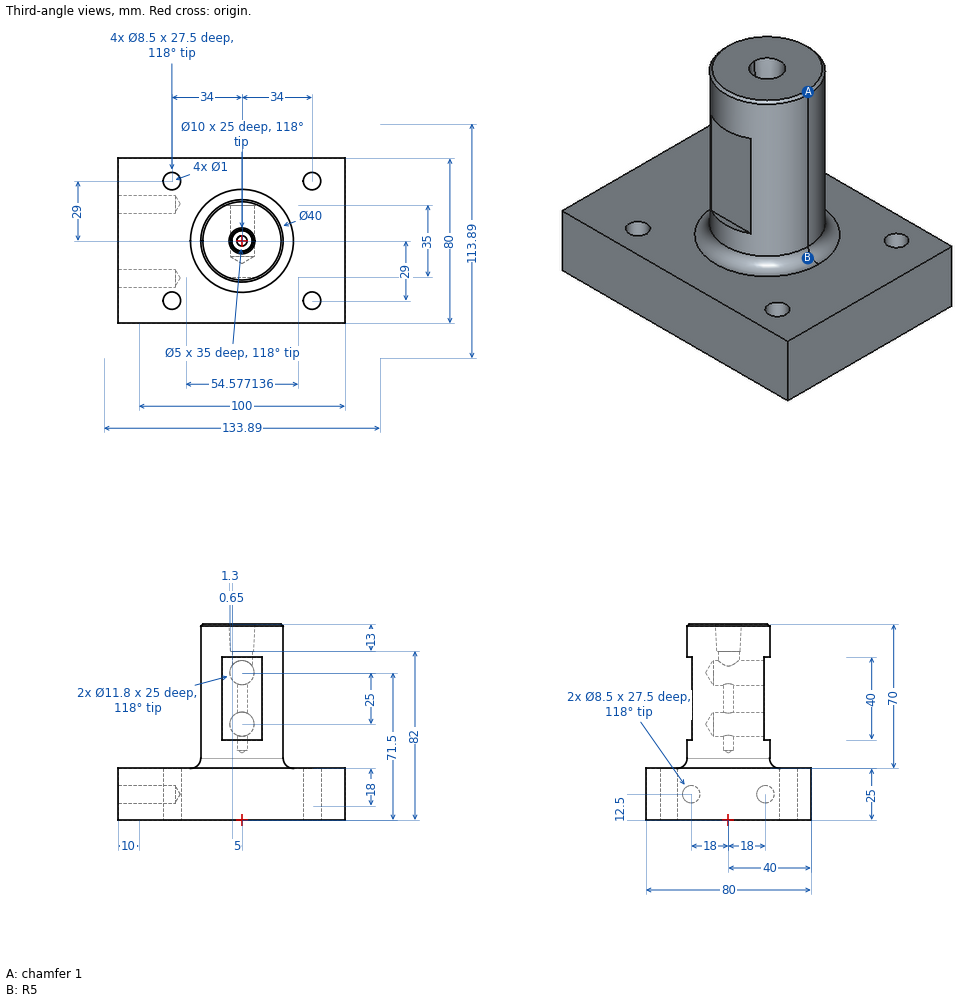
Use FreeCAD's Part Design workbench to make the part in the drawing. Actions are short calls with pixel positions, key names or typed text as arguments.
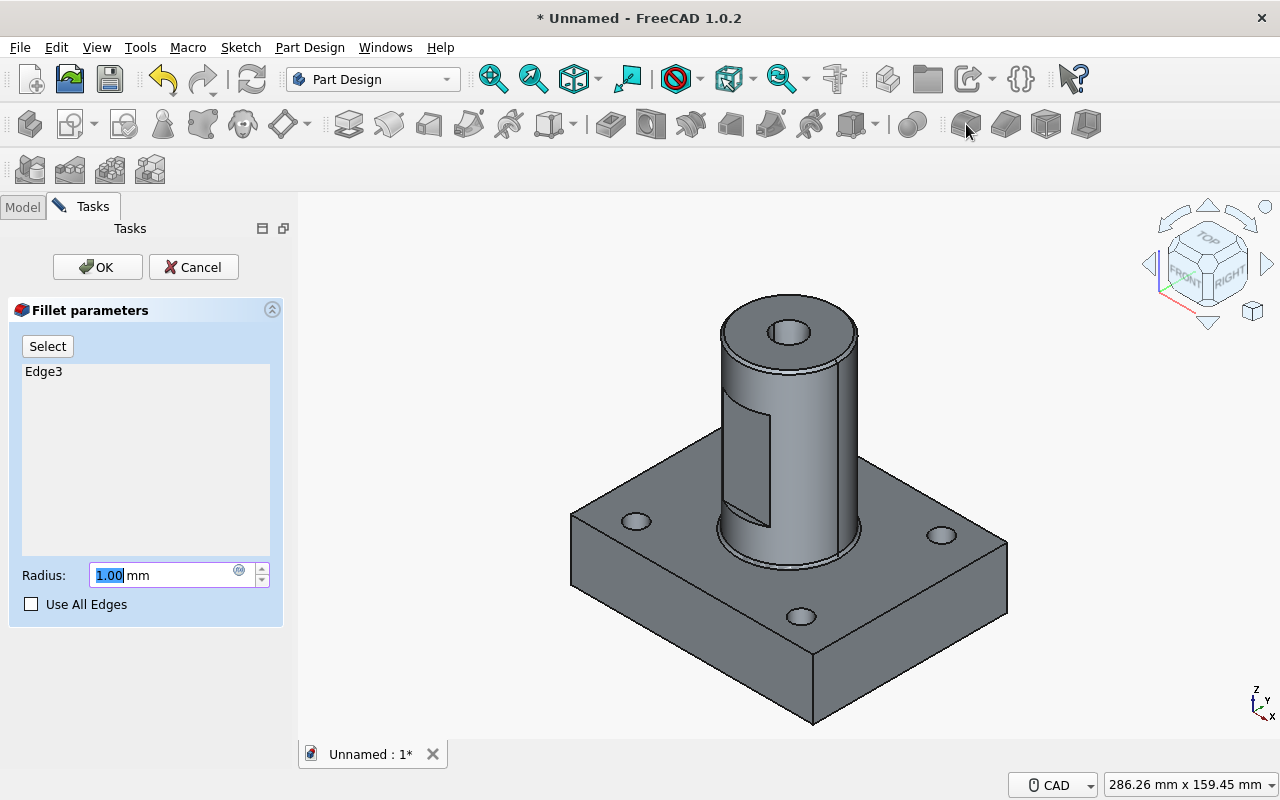
text(5)
key(Tab)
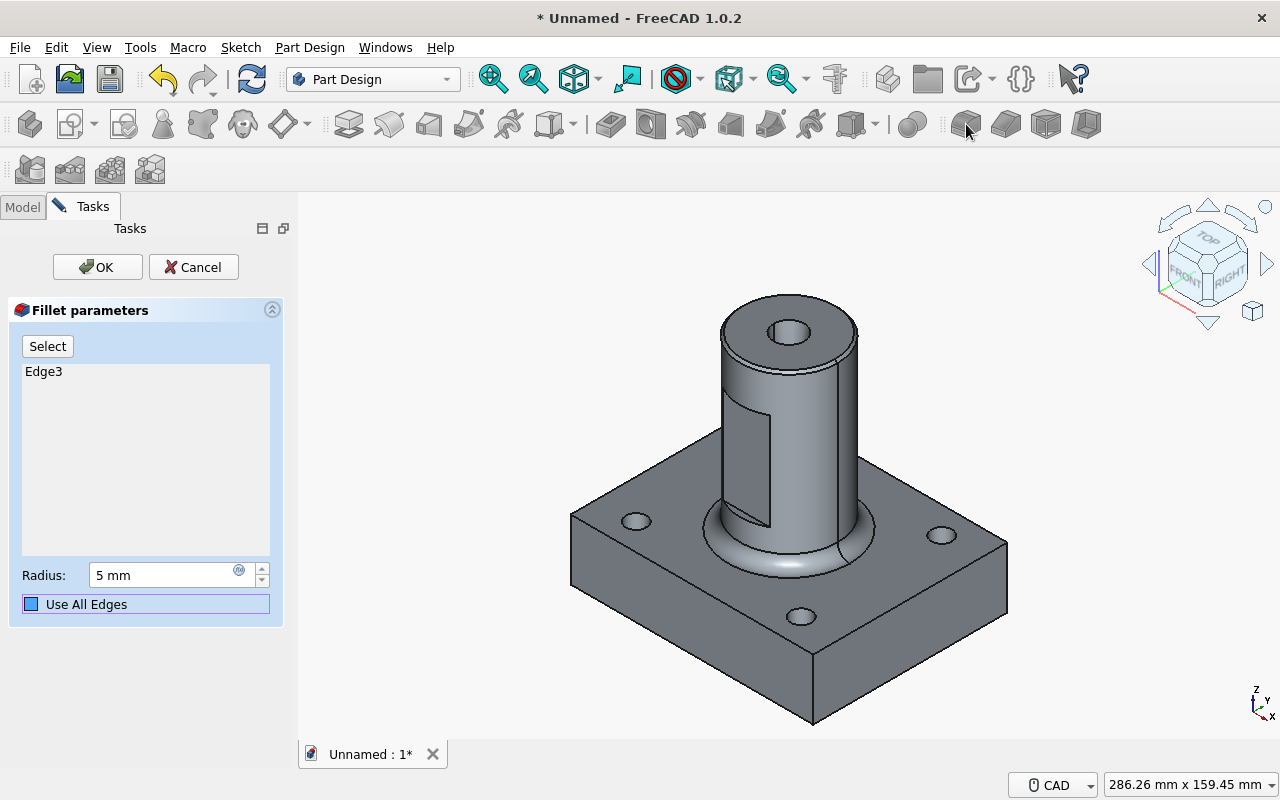
click(98, 267)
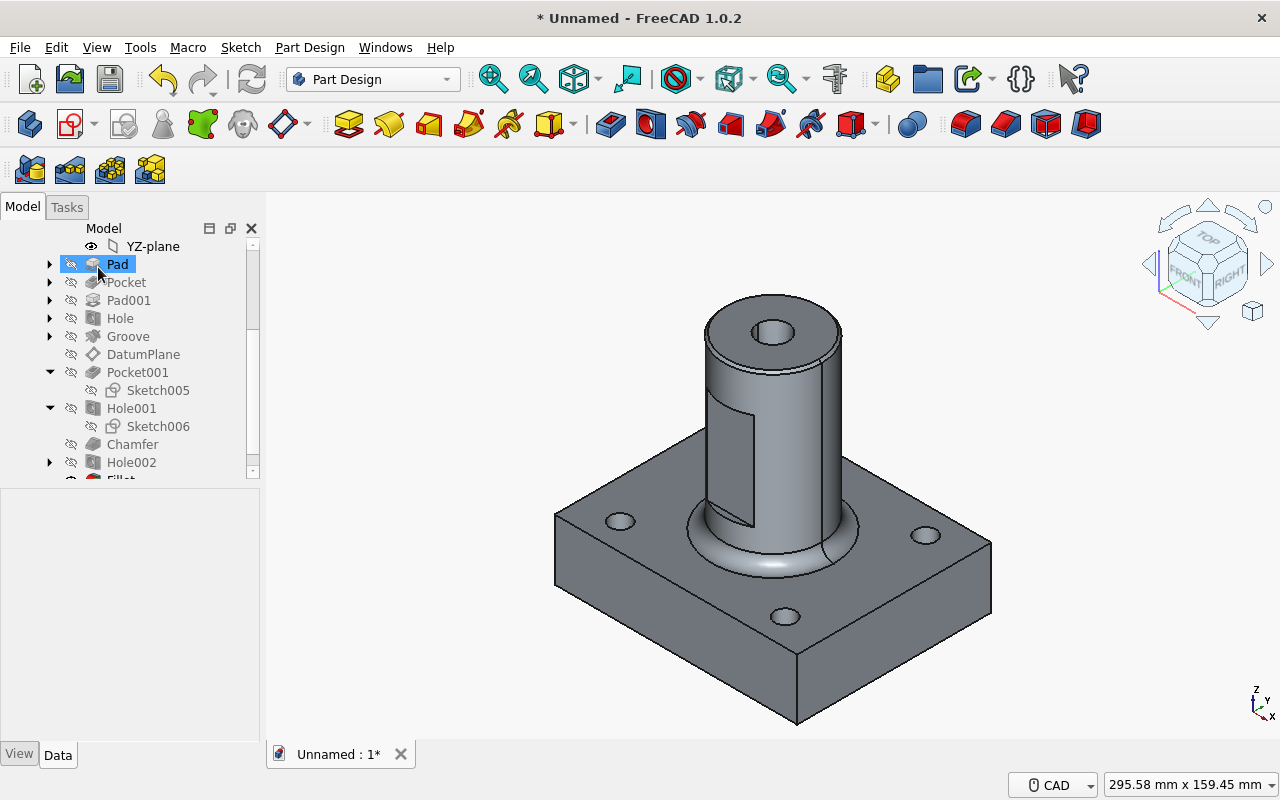
scroll(160, 350, down, 3)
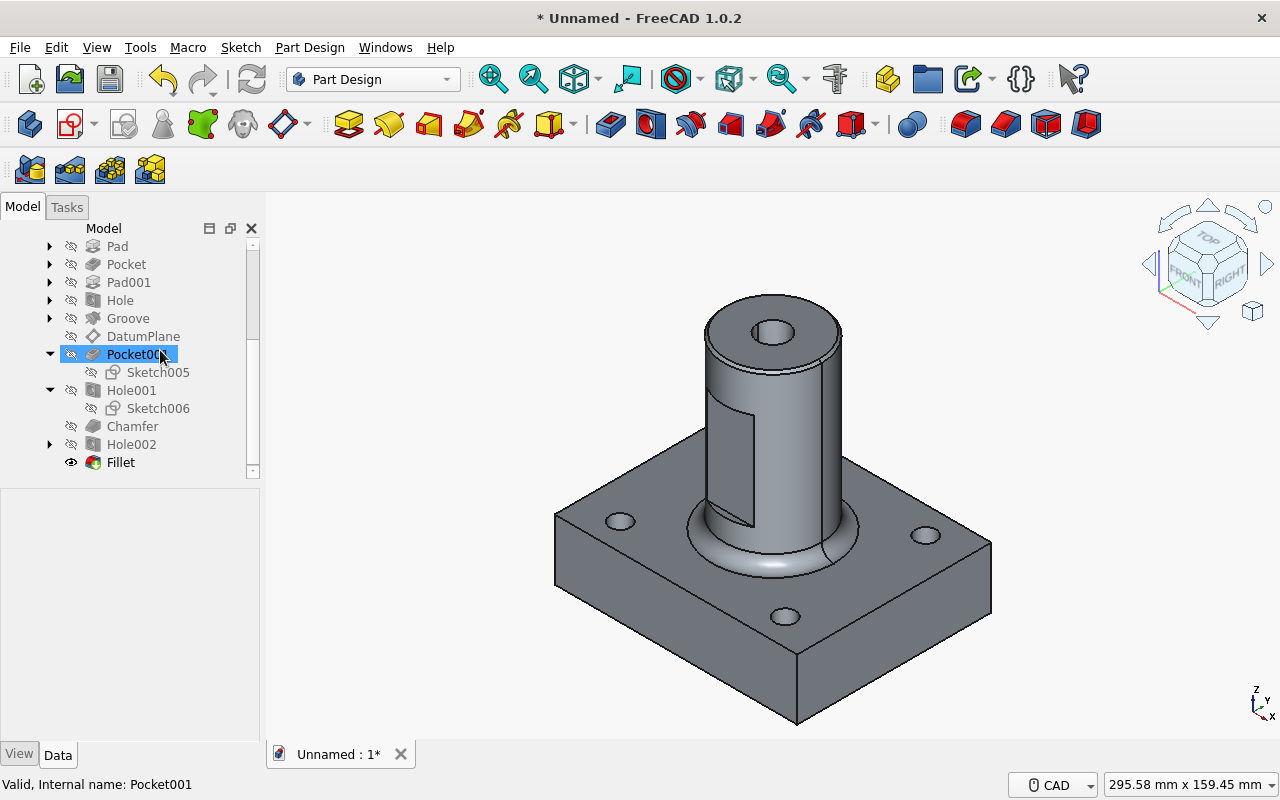
scroll(140, 350, up, 15)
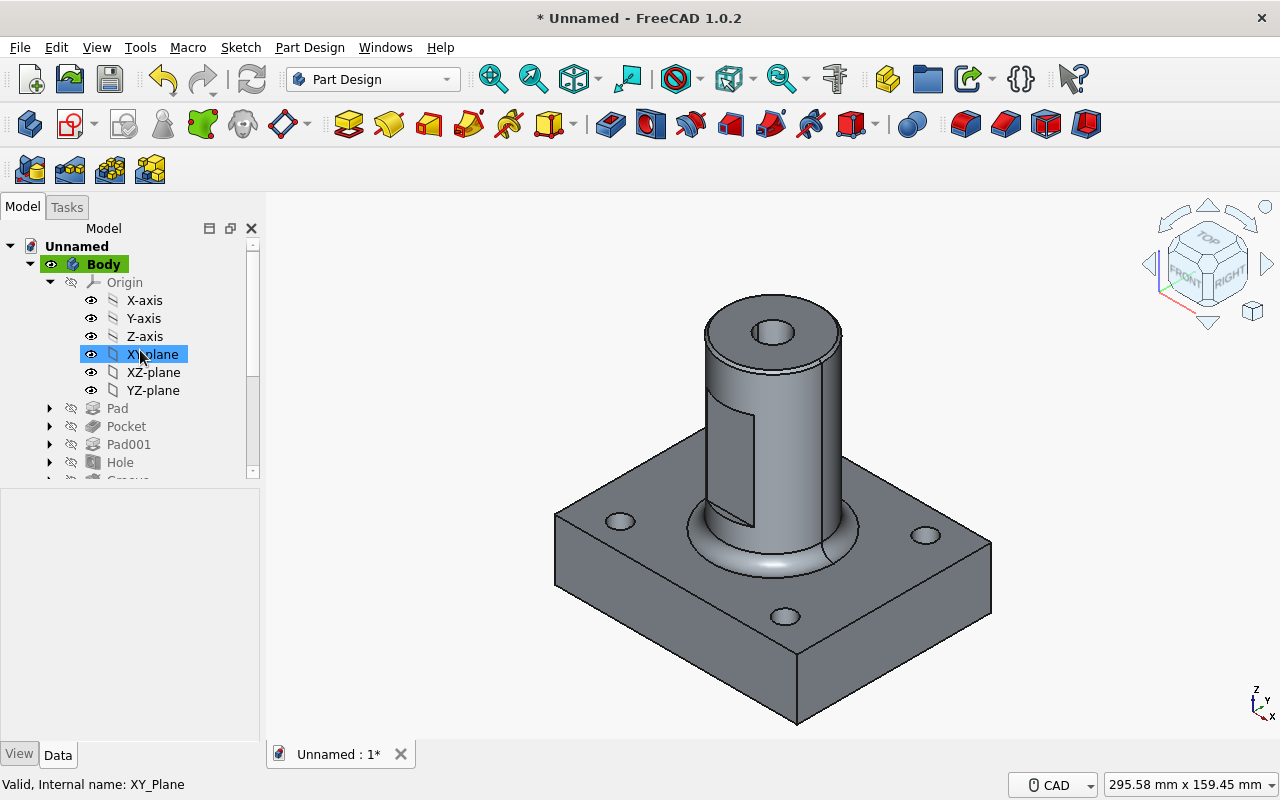
click(136, 354)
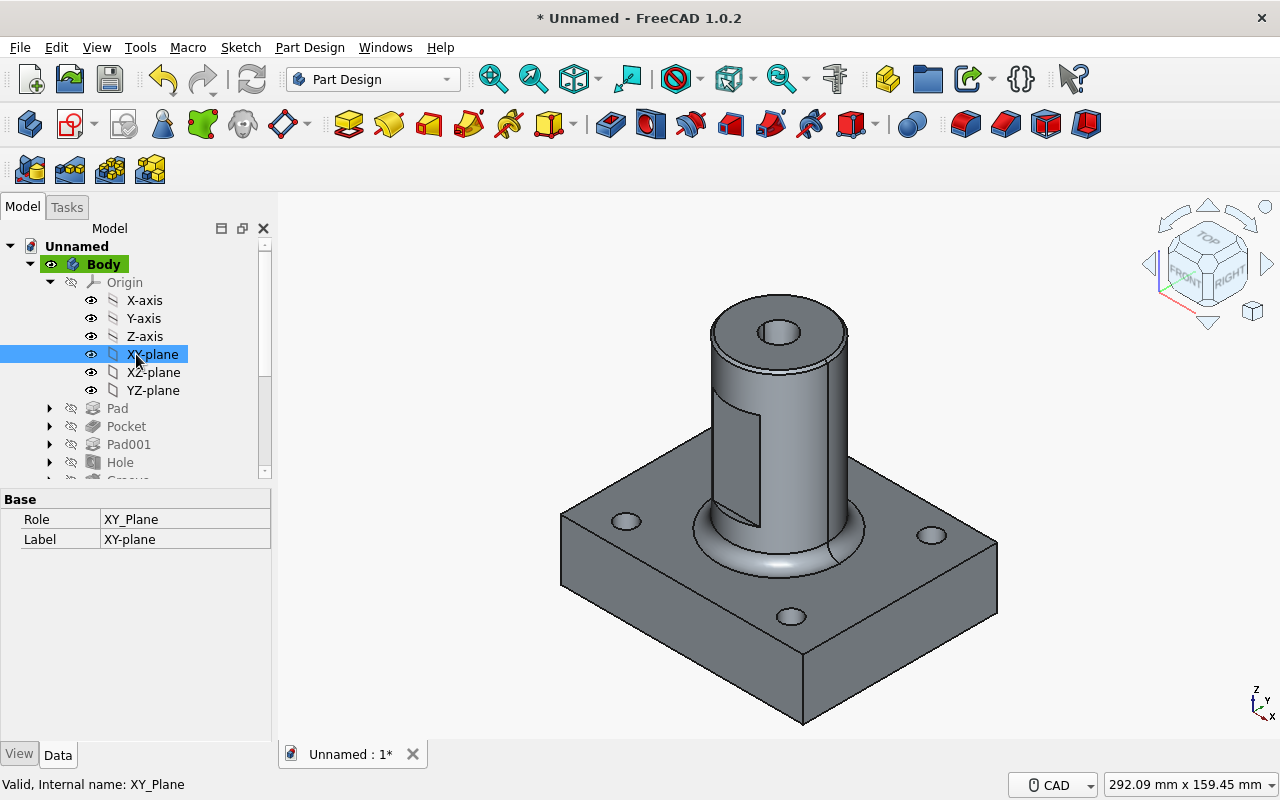
click(284, 124)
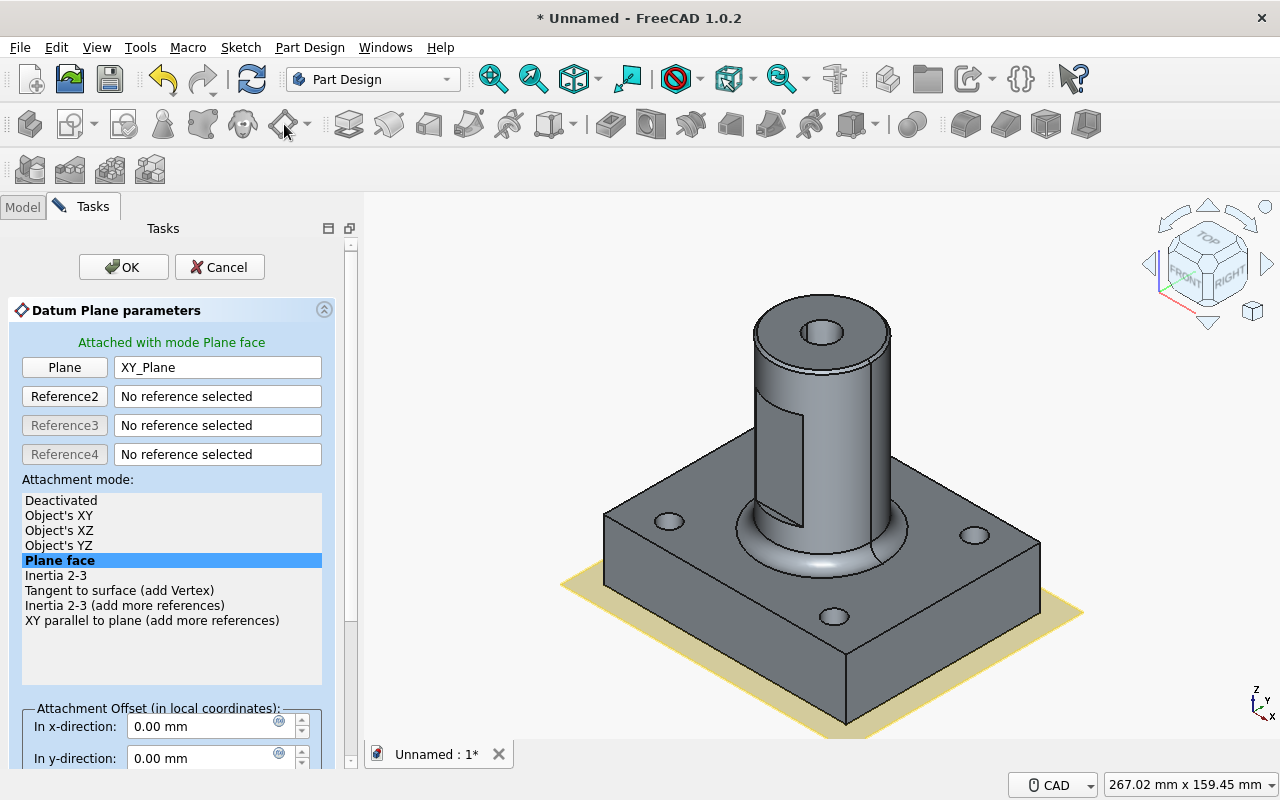
scroll(351, 503, down, 2)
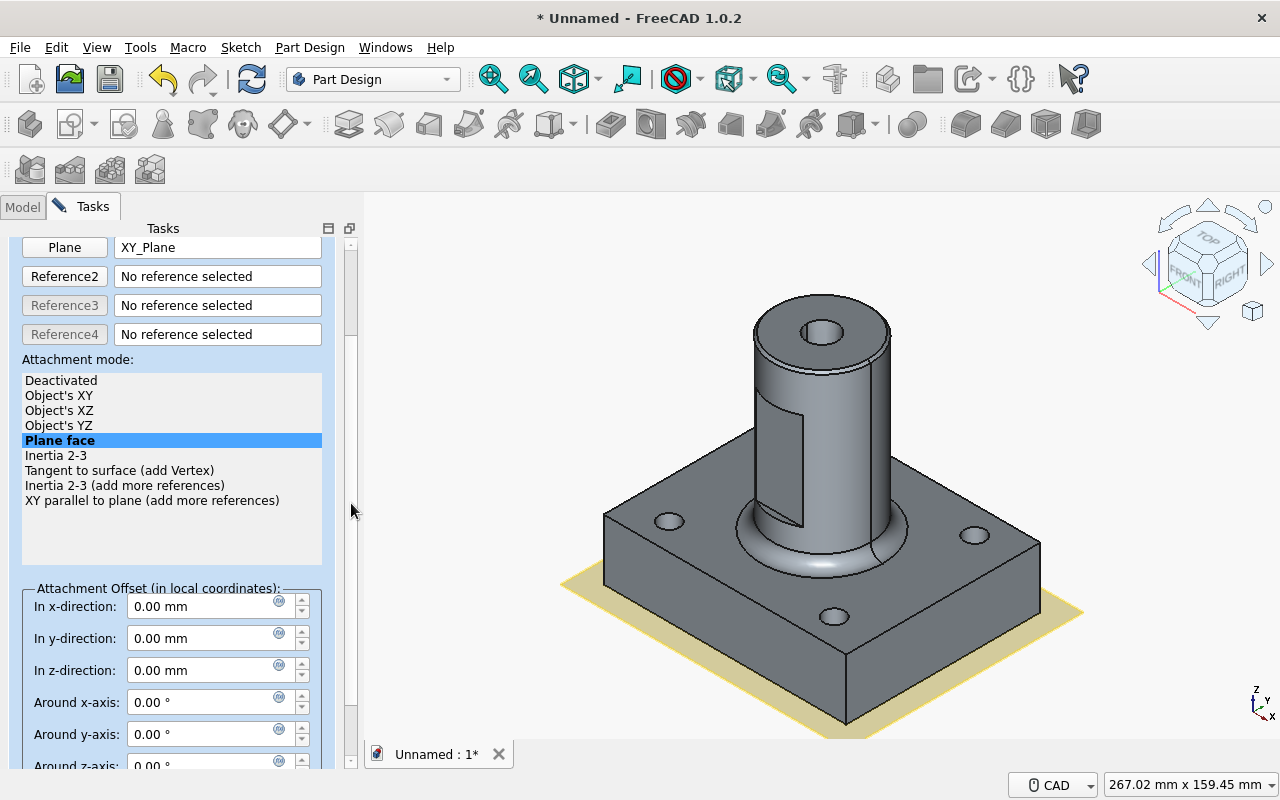
triple_click(210, 670)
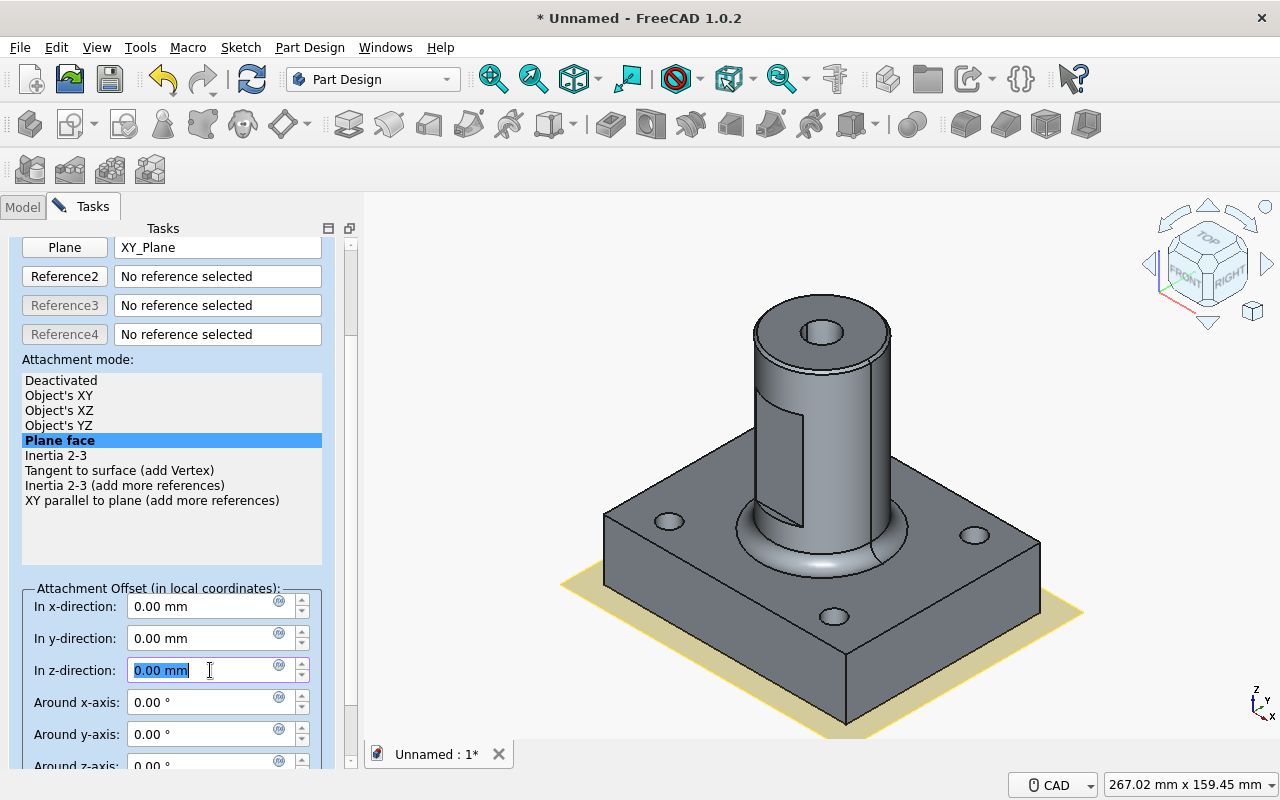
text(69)
key(Tab)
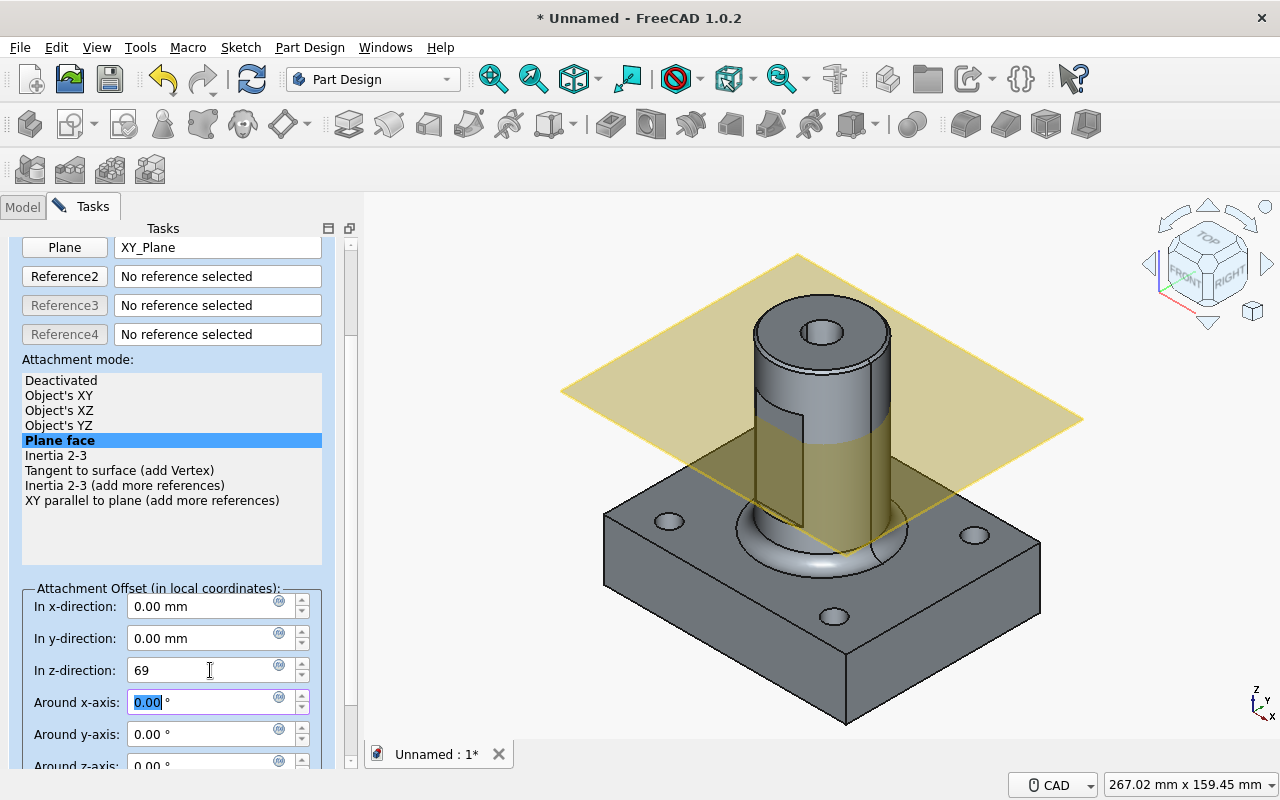
scroll(351, 503, up, 3)